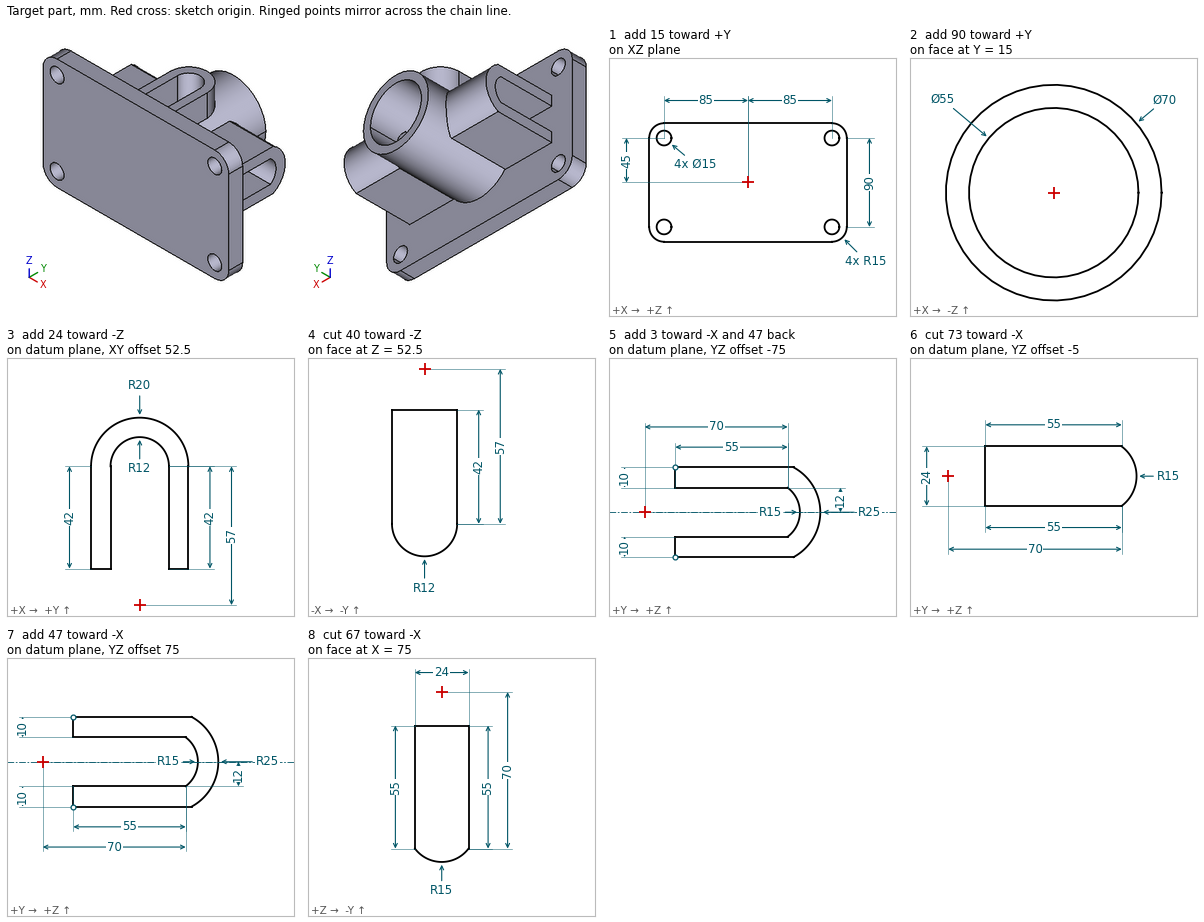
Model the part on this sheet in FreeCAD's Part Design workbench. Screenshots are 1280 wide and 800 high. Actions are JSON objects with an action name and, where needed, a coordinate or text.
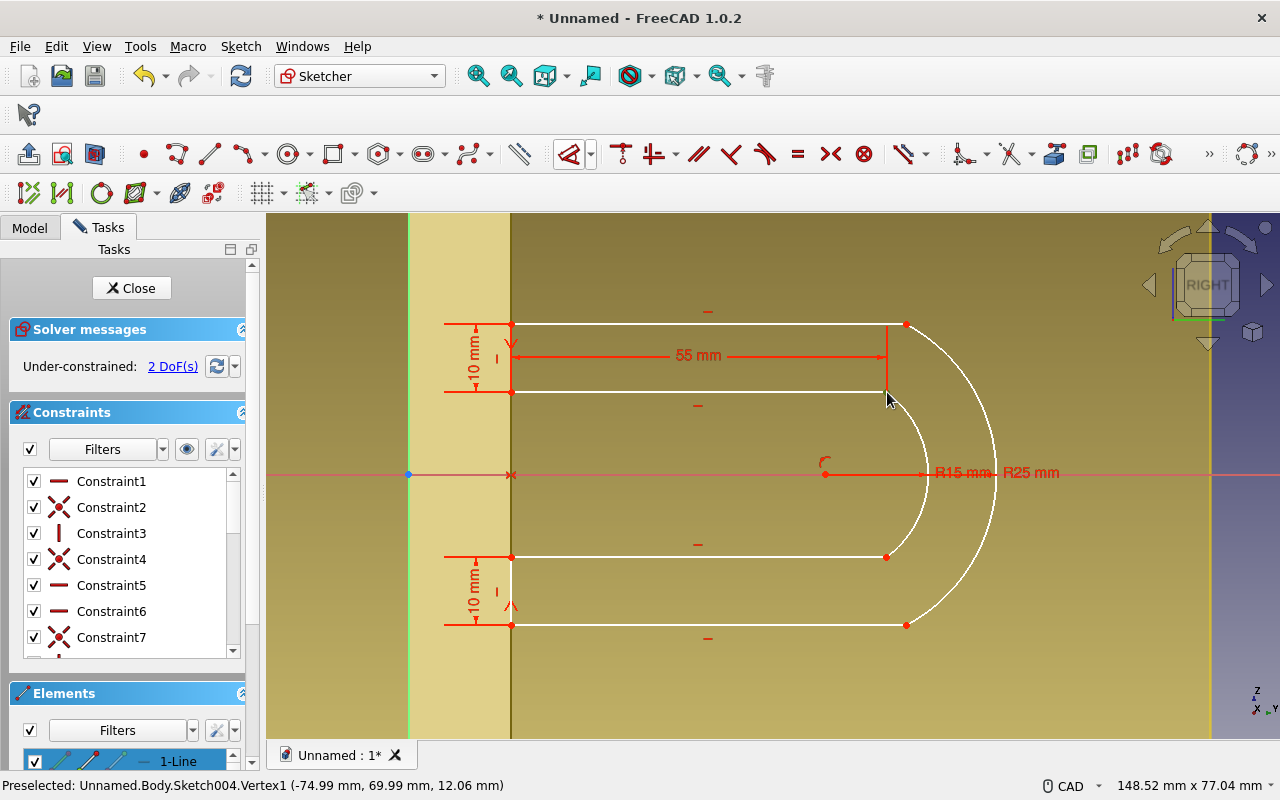
{"action": "key", "text": "l"}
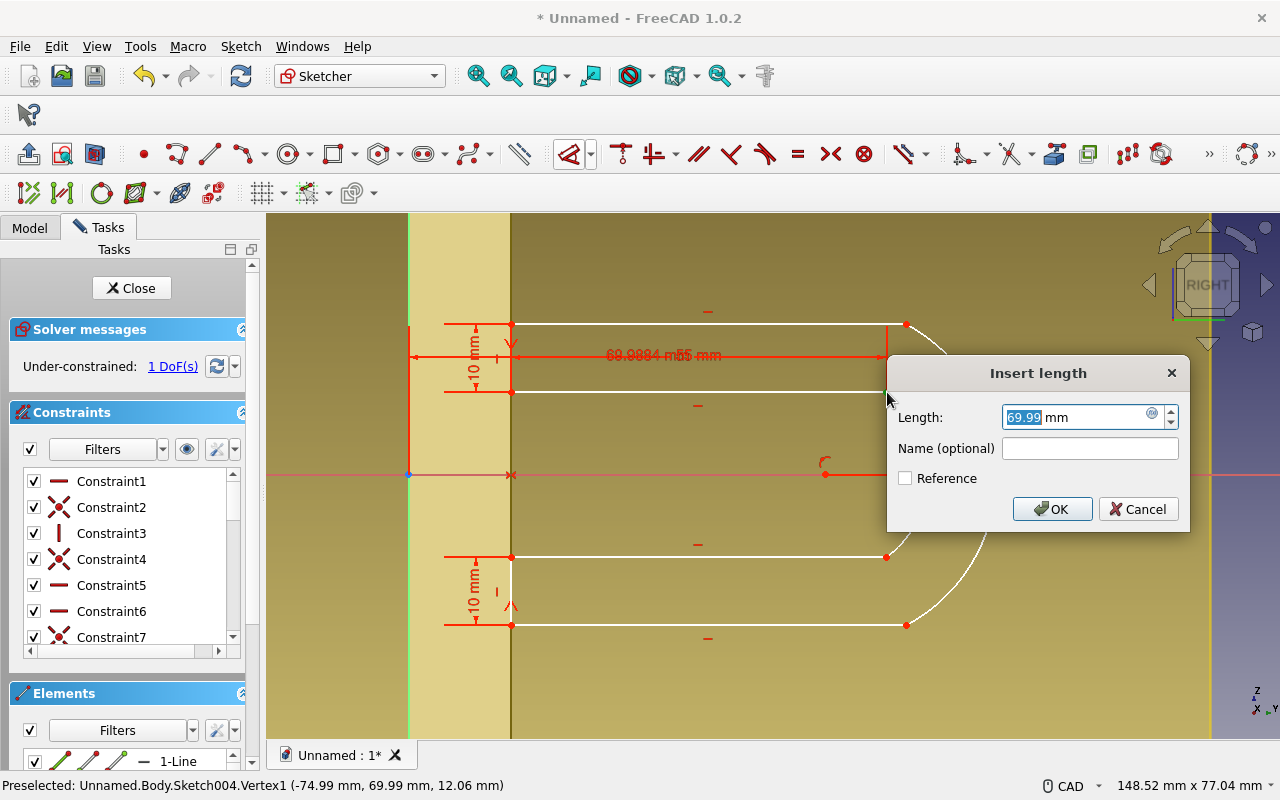
{"action": "type", "text": "70"}
{"action": "key", "text": "Return"}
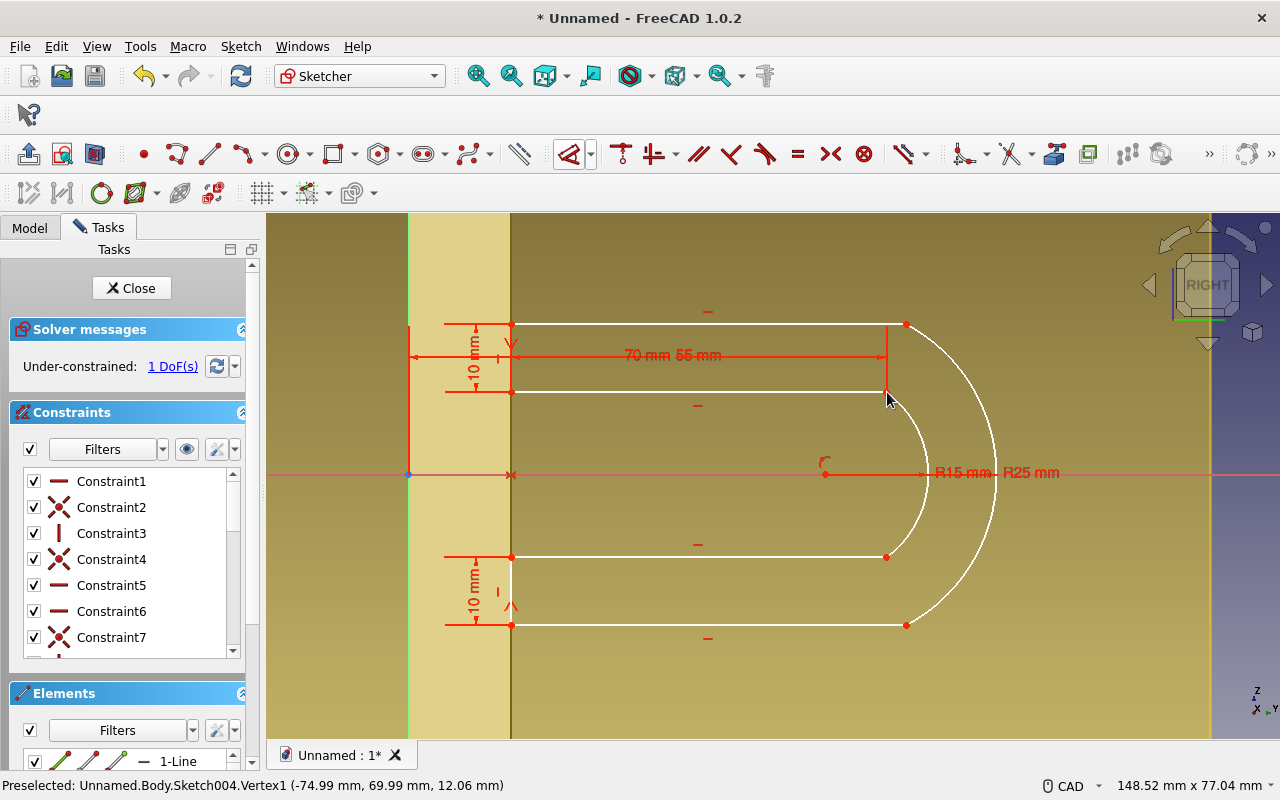
{"action": "left_click", "coordinate": [887, 392]}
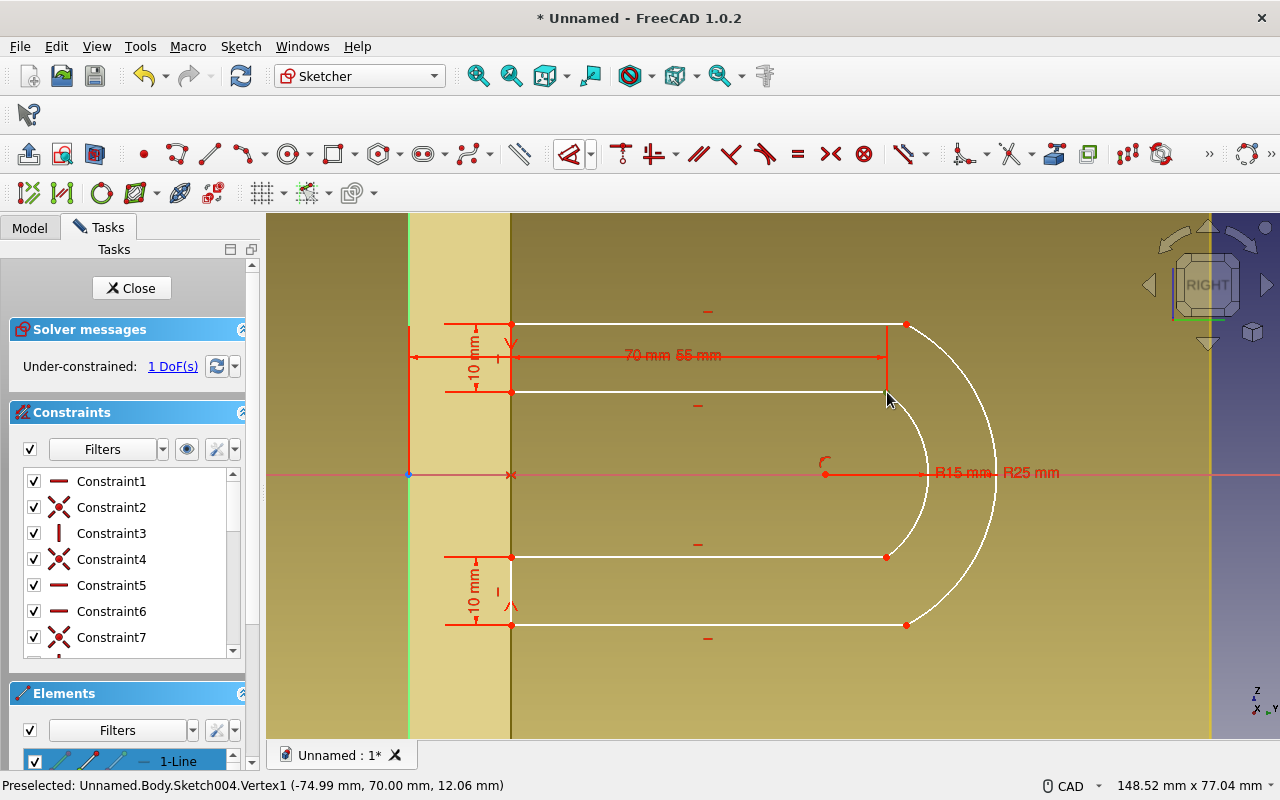
{"action": "key", "text": "i"}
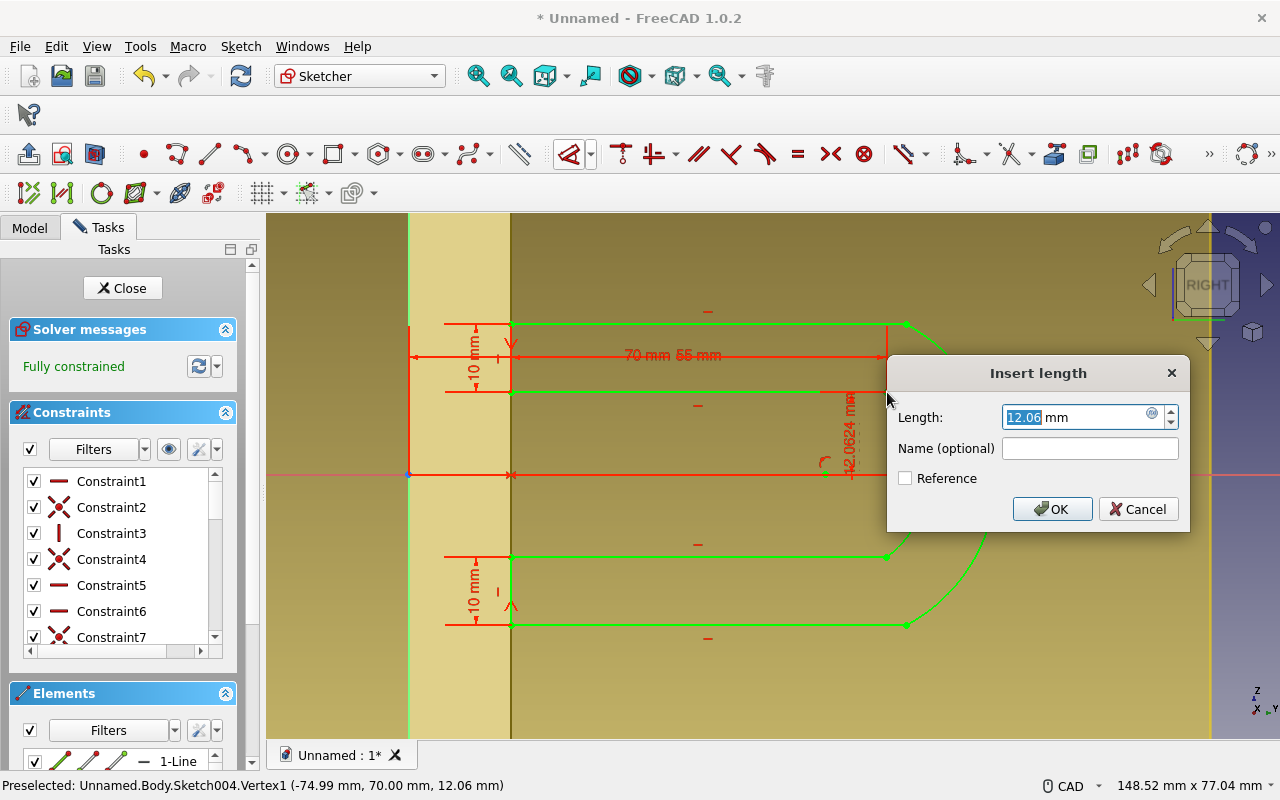
{"action": "type", "text": "12"}
{"action": "key", "text": "Return"}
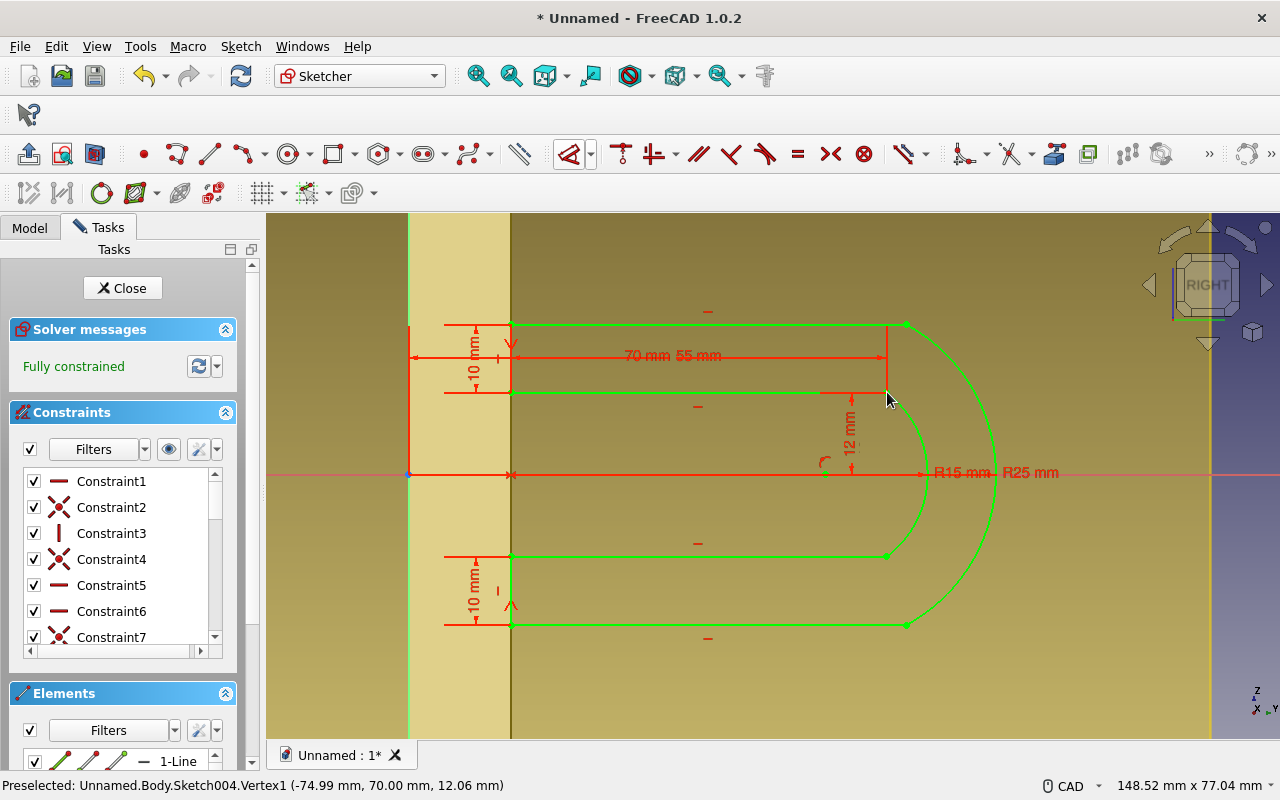
{"action": "left_click", "coordinate": [123, 288]}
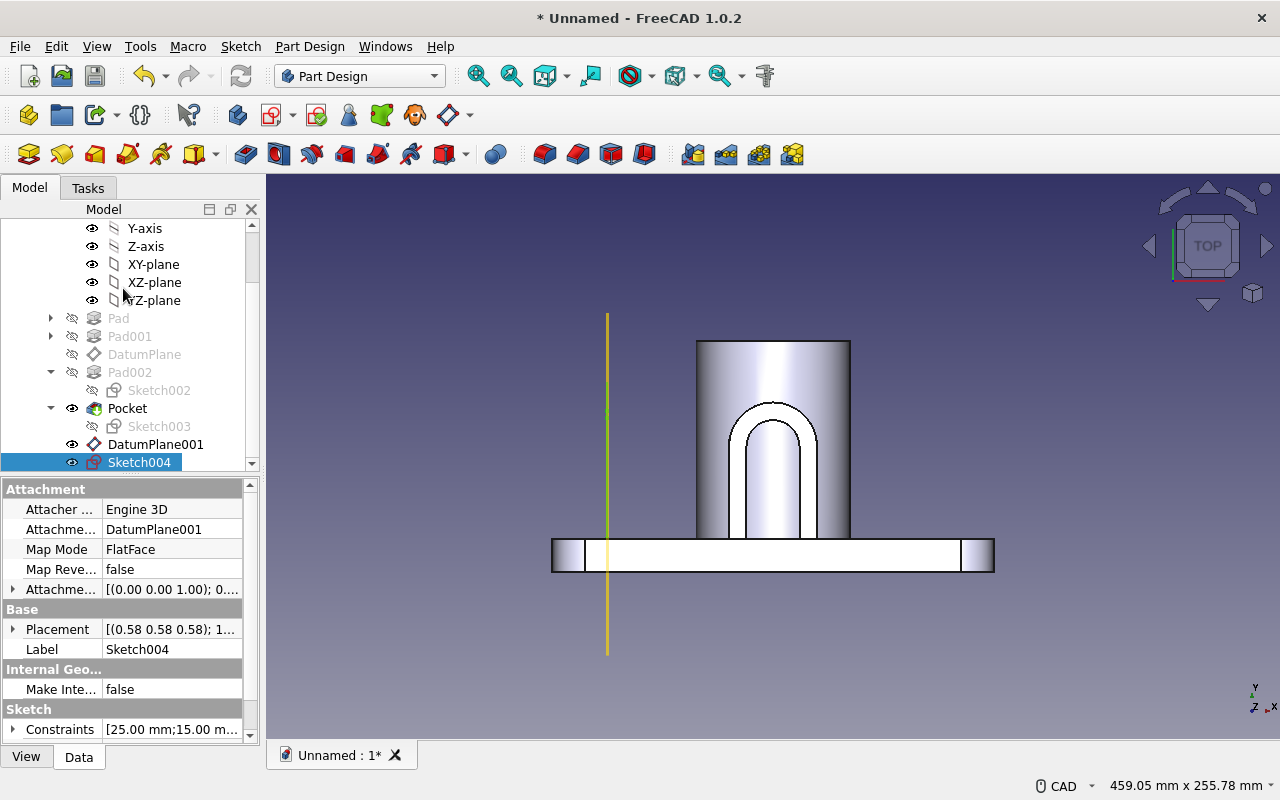
{"action": "left_click", "coordinate": [29, 154]}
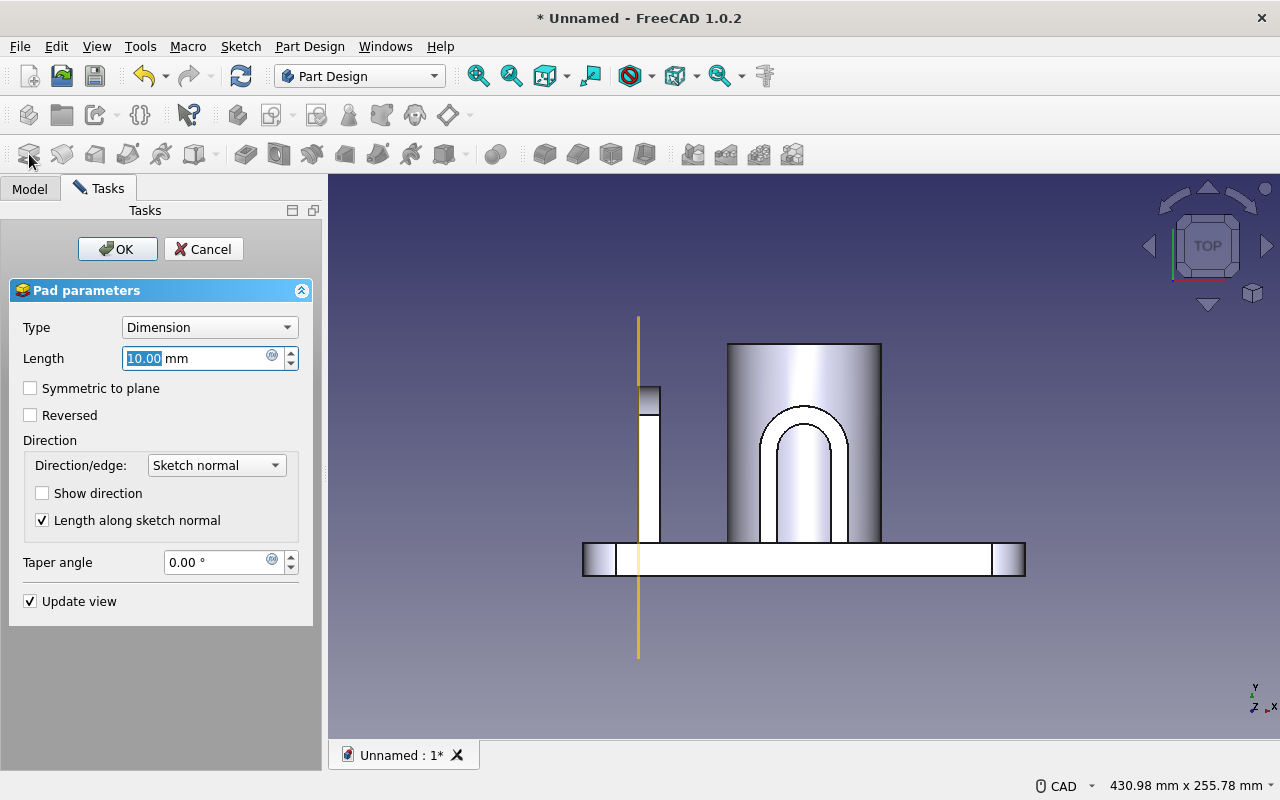
{"action": "left_click", "coordinate": [210, 328]}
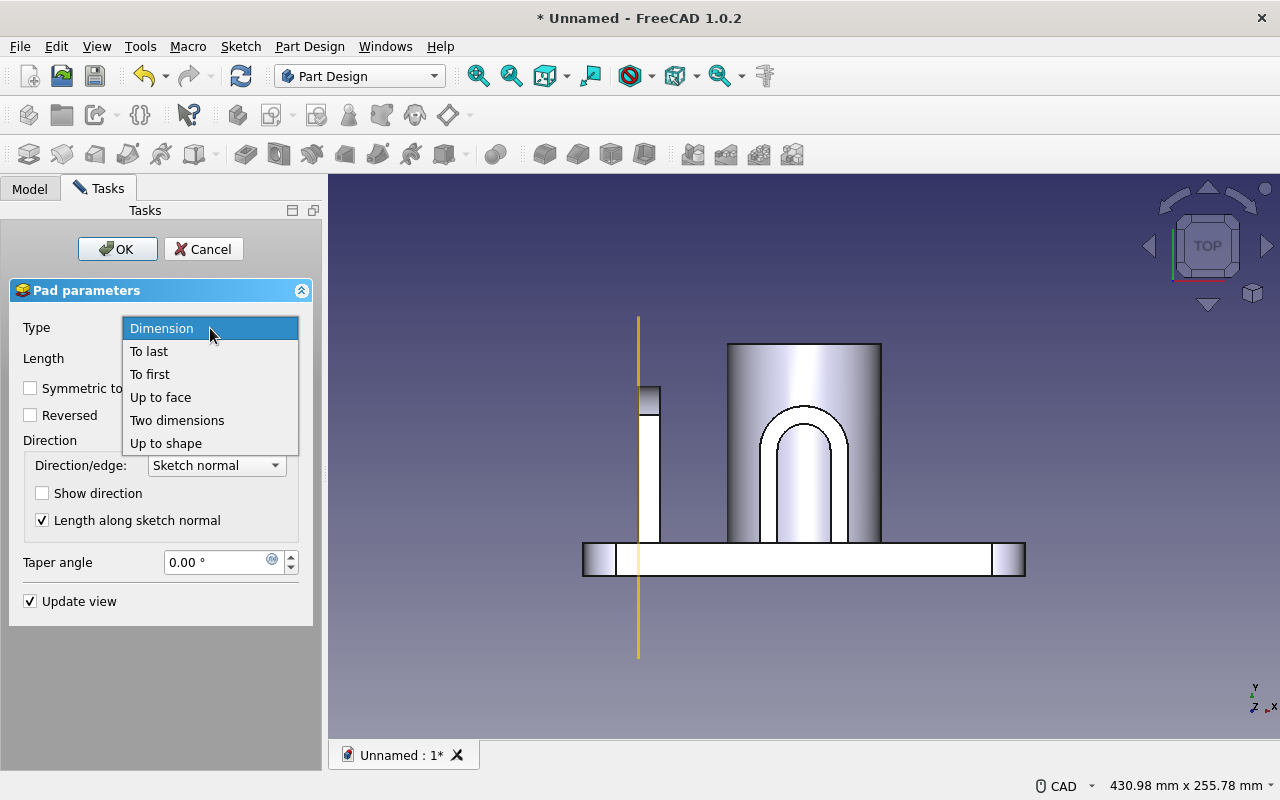
{"action": "left_click", "coordinate": [208, 420]}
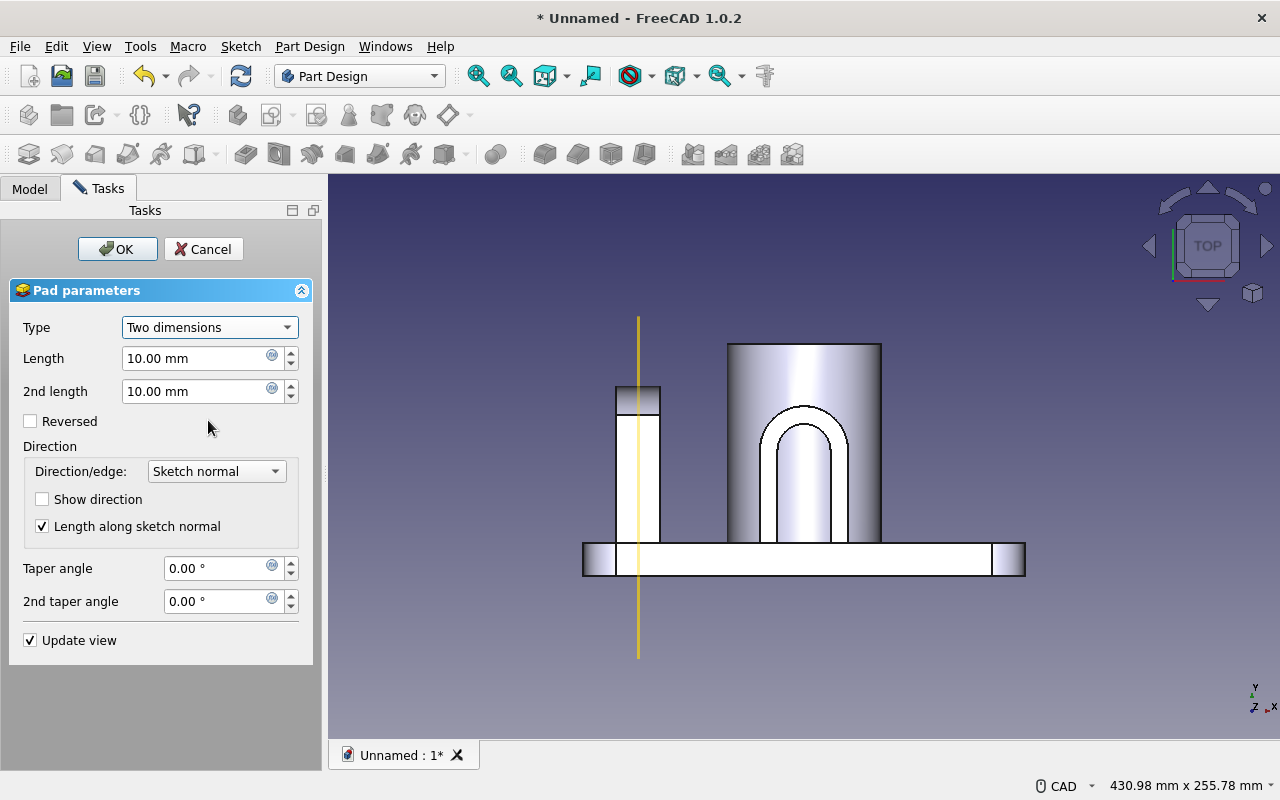
{"action": "triple_click", "coordinate": [204, 358]}